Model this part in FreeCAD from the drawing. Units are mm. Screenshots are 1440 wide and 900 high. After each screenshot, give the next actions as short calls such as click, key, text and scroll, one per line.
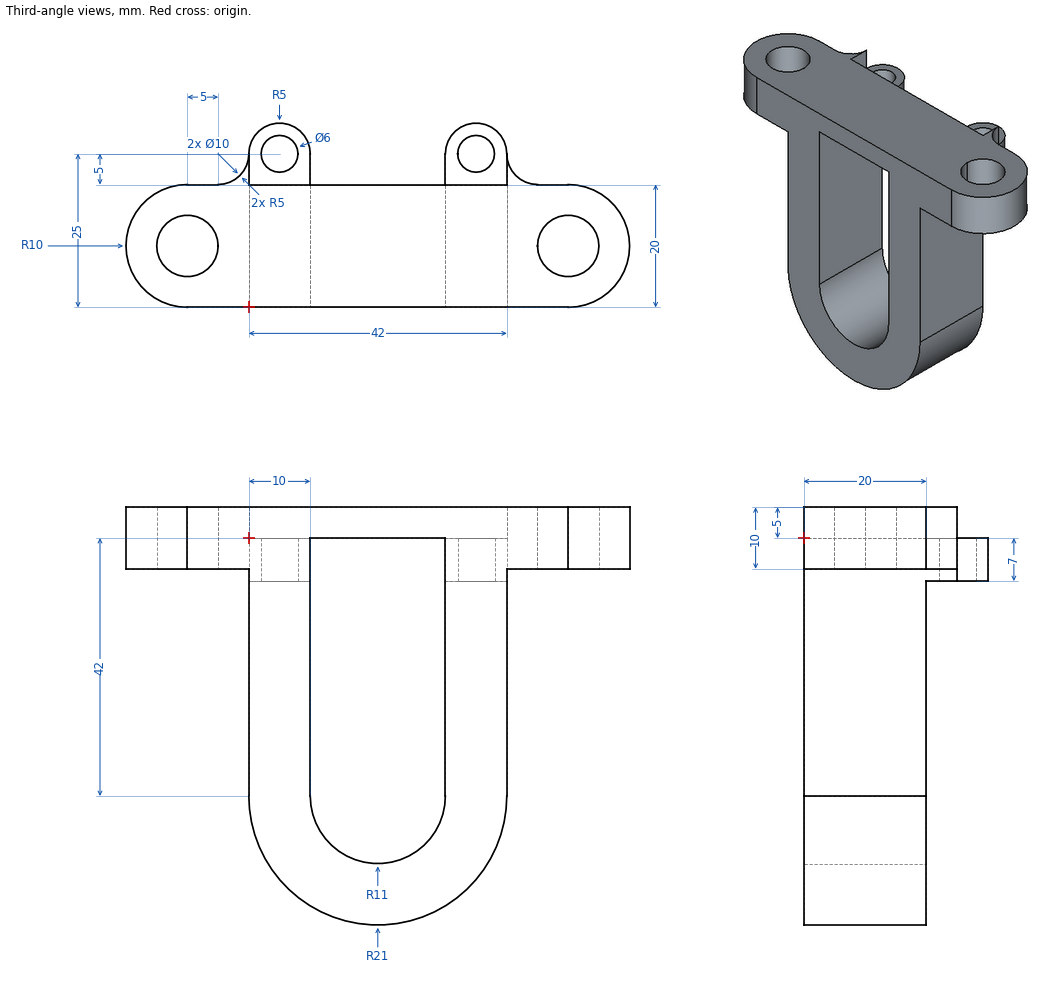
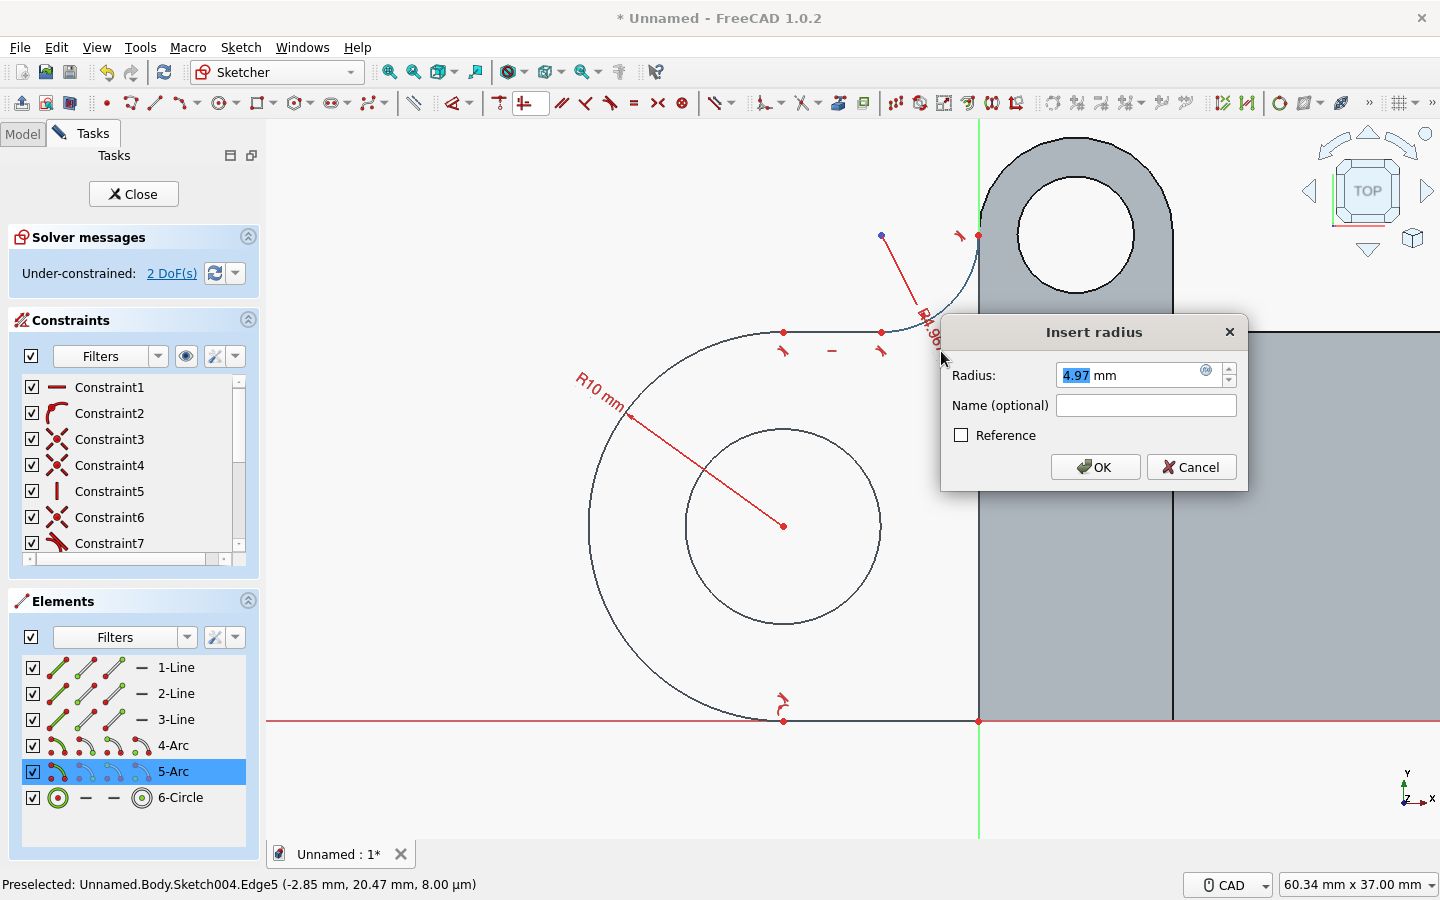
text(5)
key(Return)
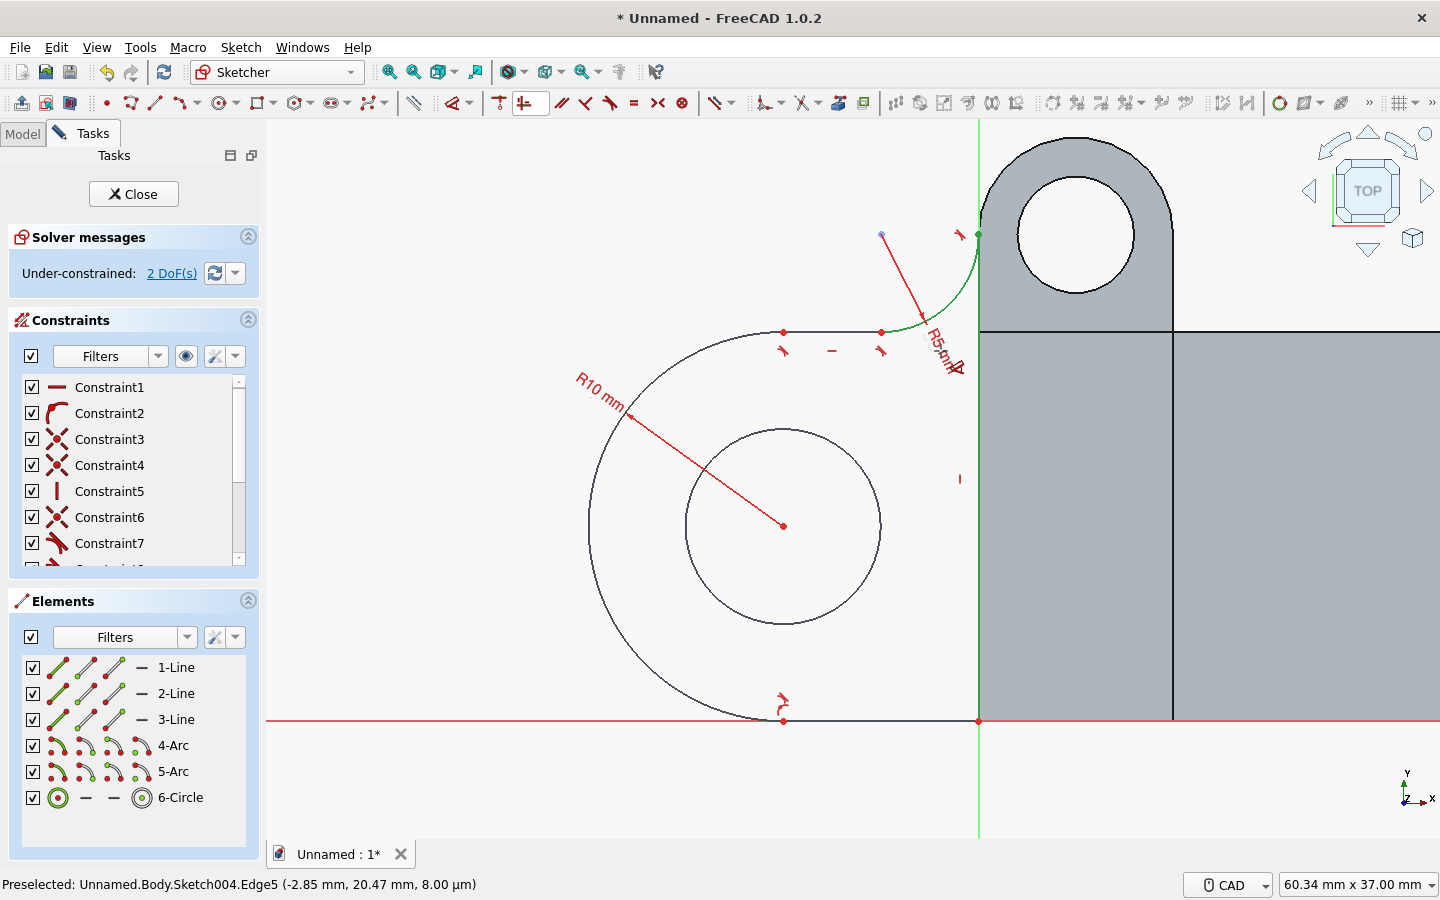
click(852, 457)
click(875, 434)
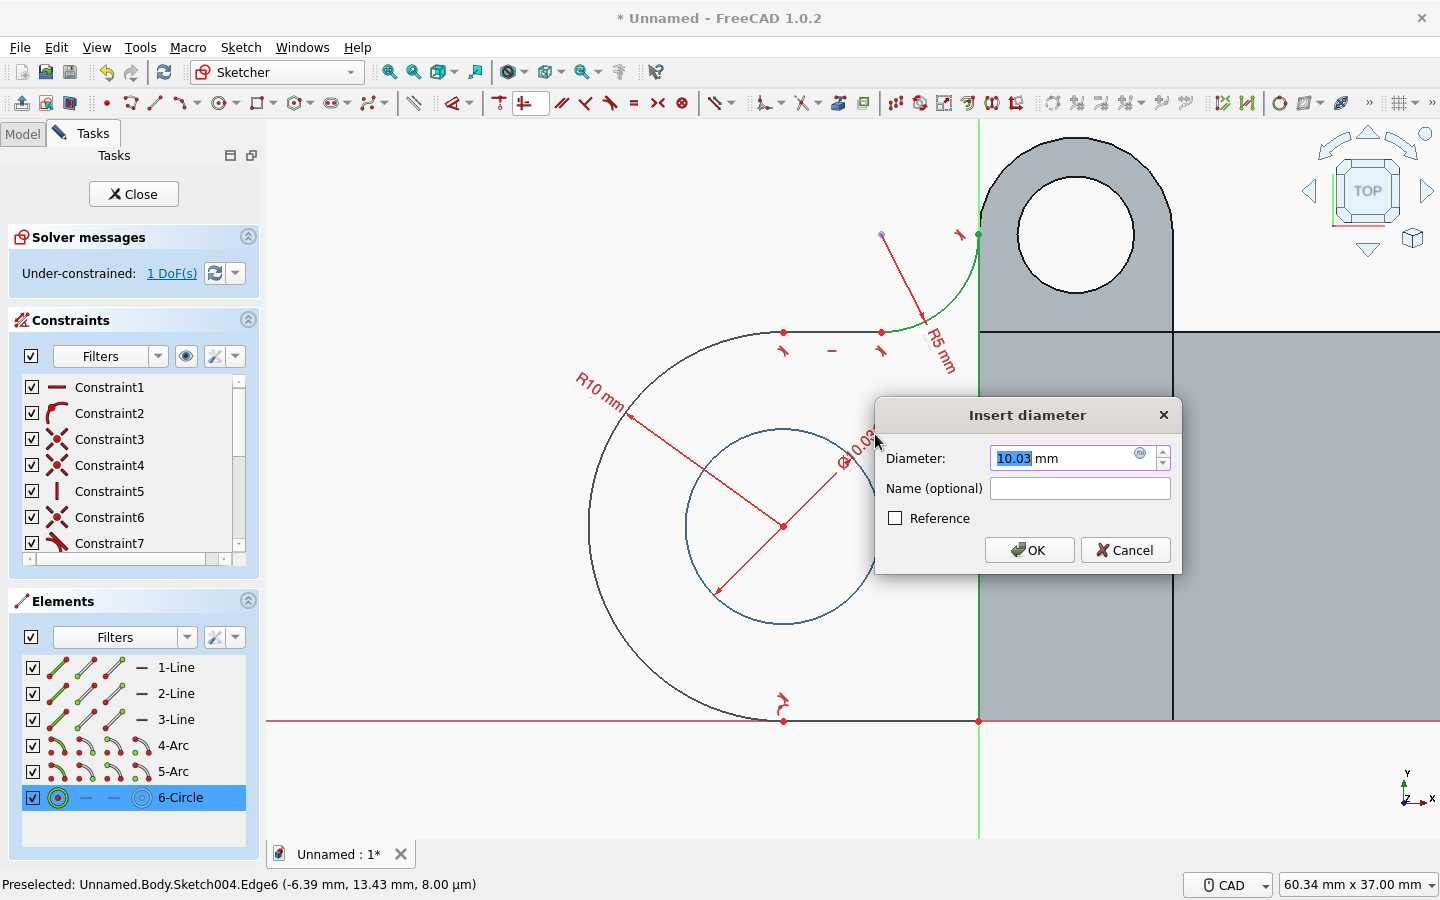
text(10)
key(Return)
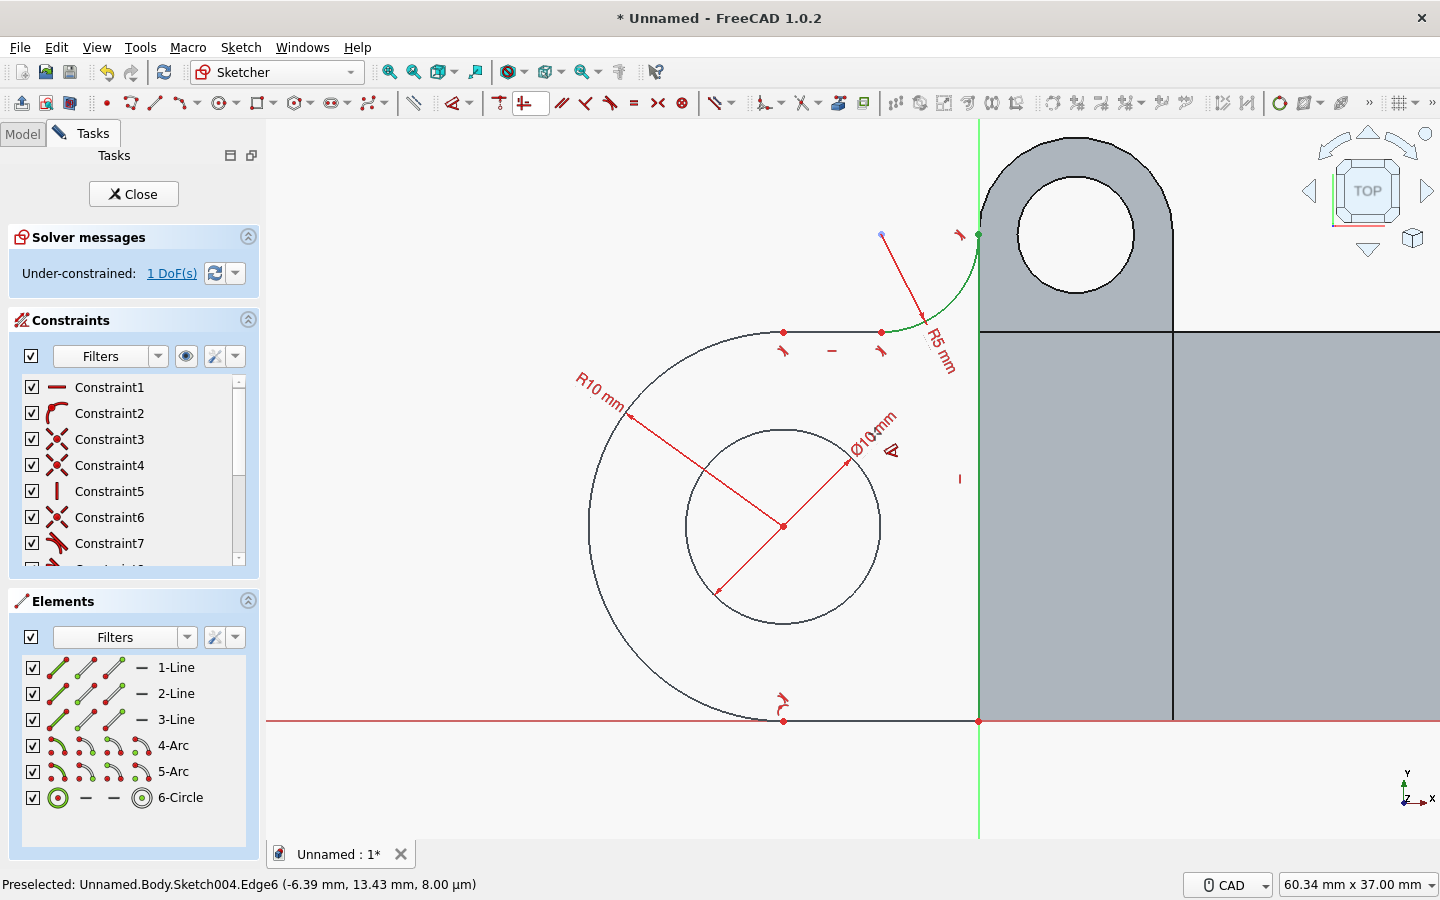
click(852, 332)
click(832, 298)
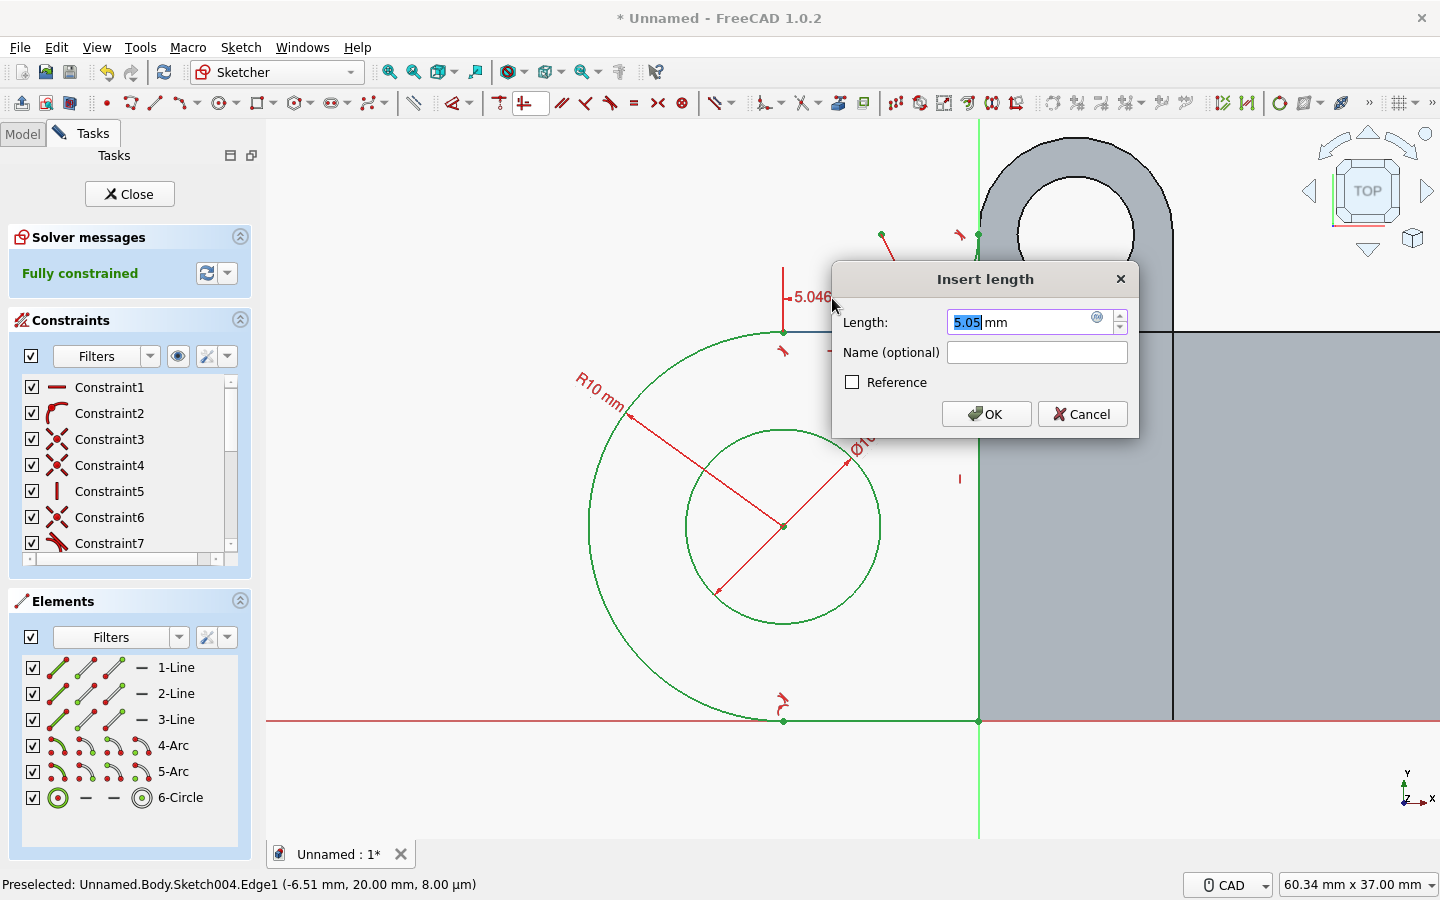
text(5)
key(Return)
key(Escape)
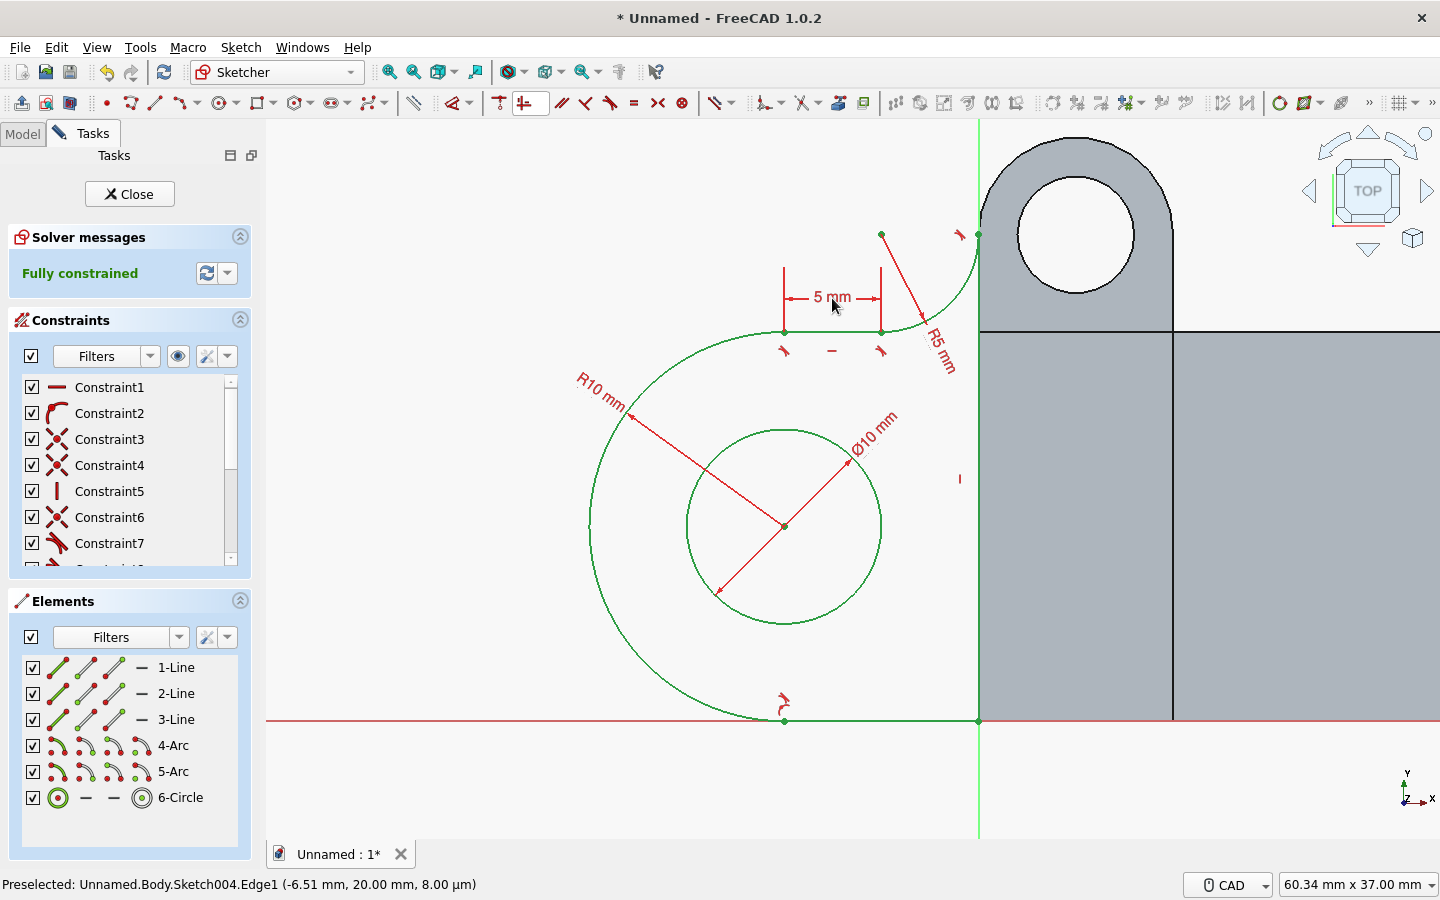
click(130, 194)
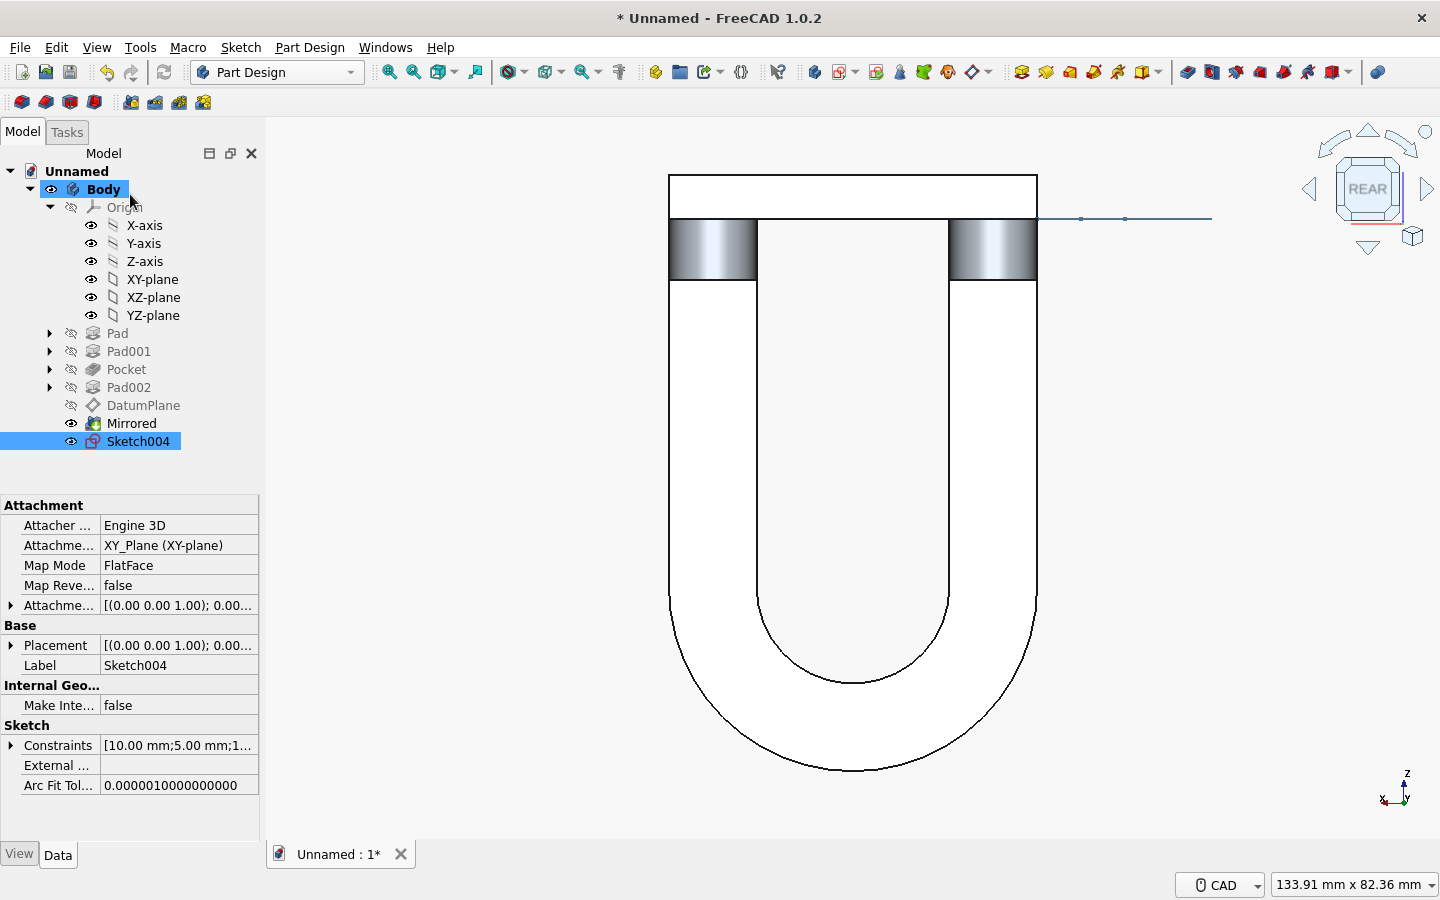
click(1022, 72)